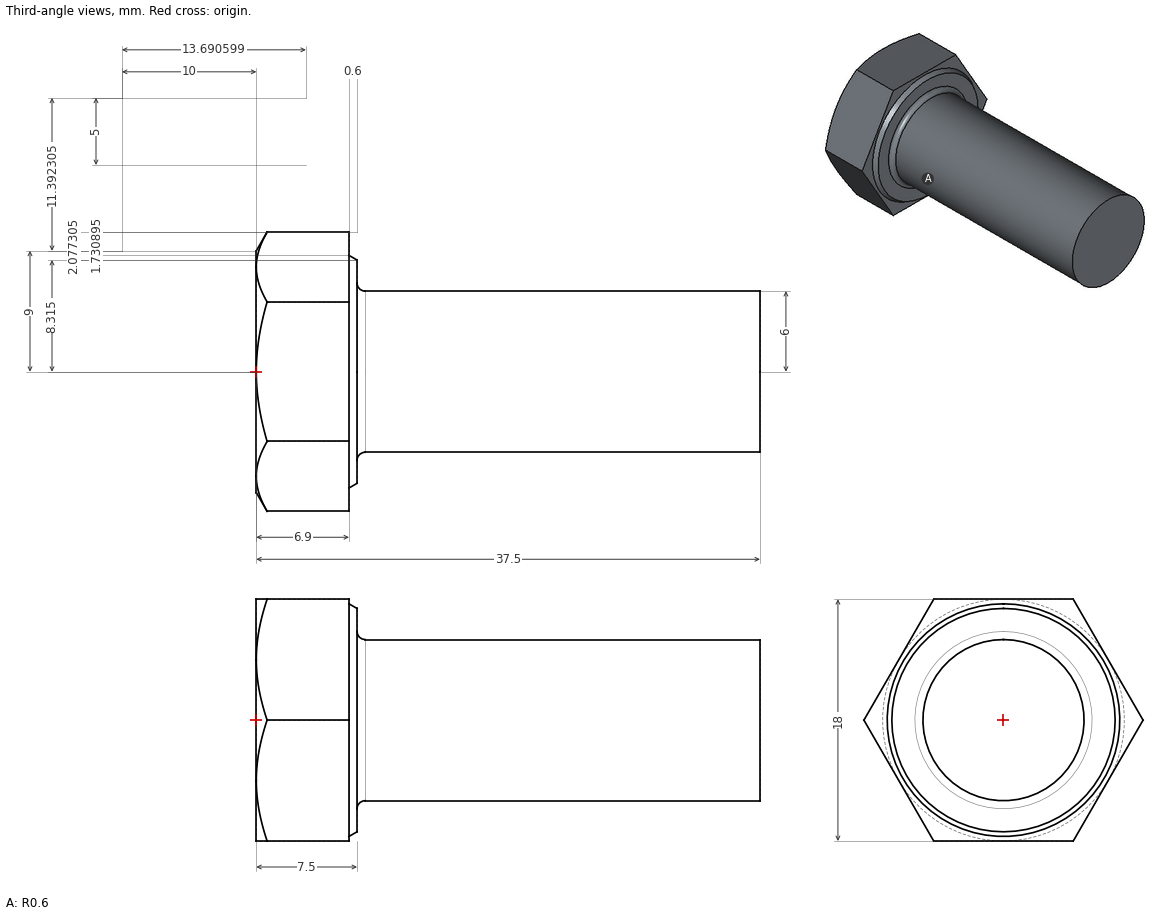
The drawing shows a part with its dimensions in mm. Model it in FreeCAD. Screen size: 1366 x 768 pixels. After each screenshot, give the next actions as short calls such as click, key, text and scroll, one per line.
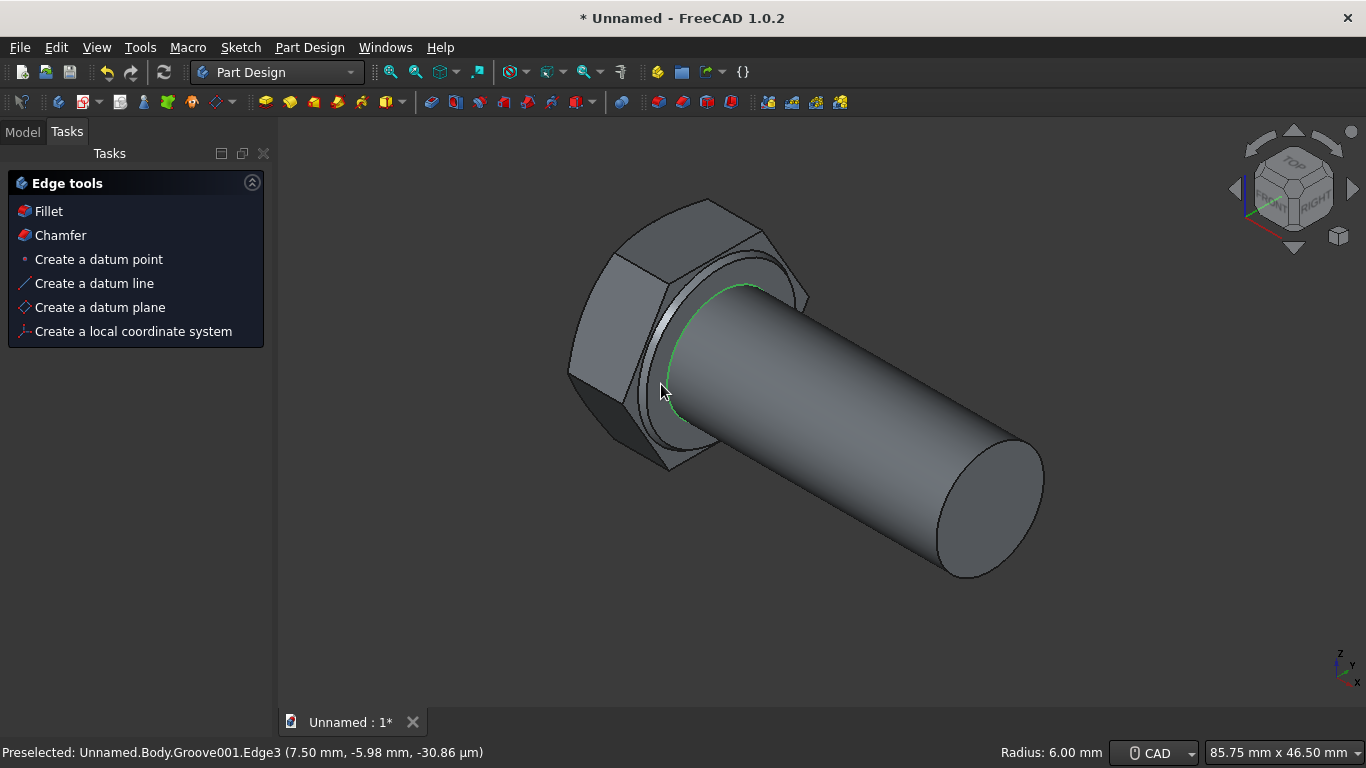
click(660, 102)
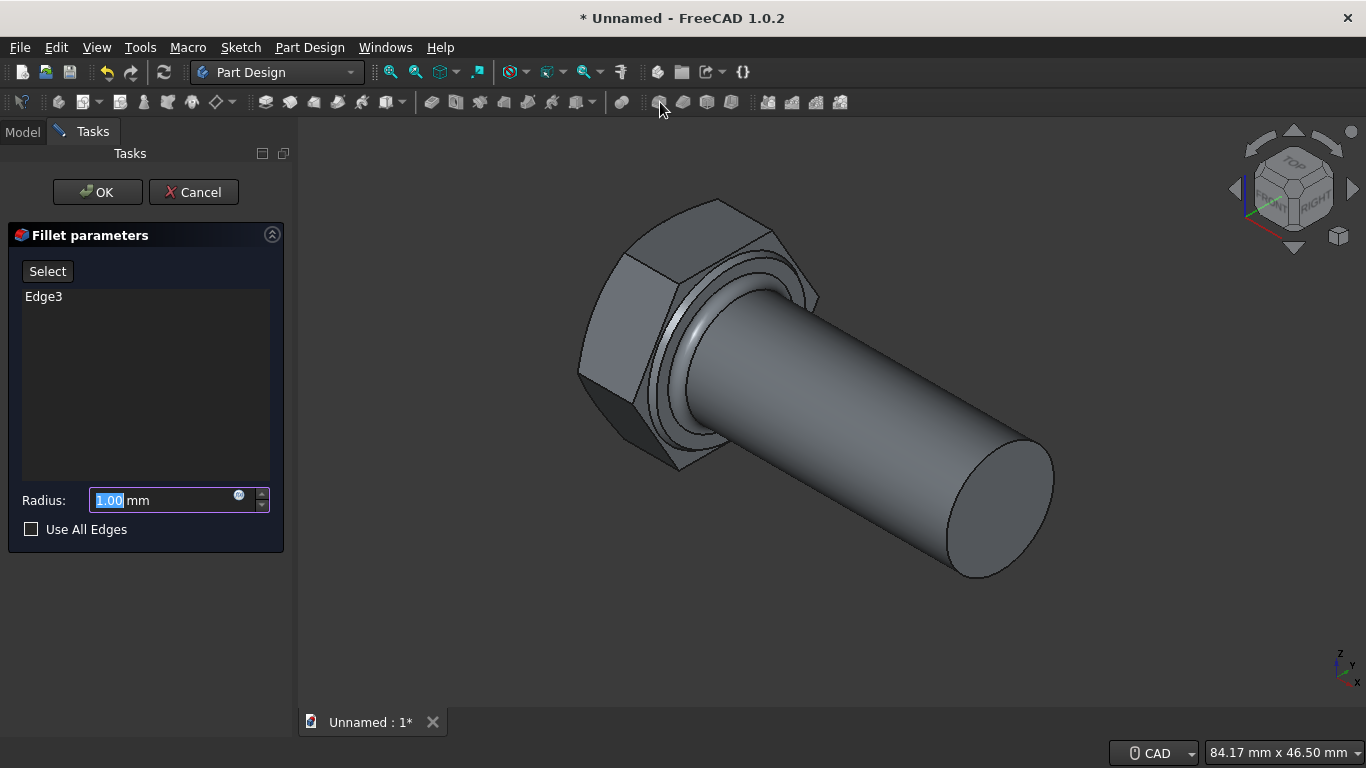
text(0.6)
key(Tab)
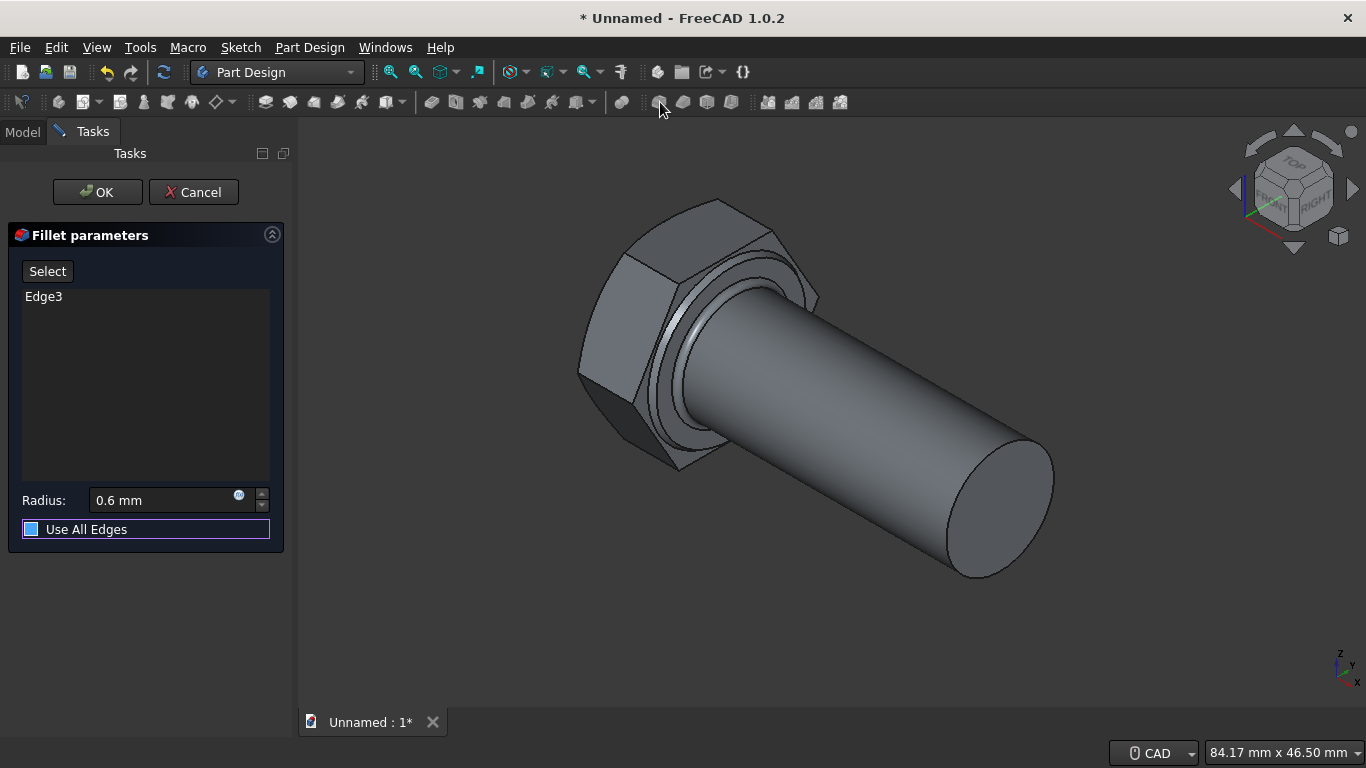
click(98, 192)